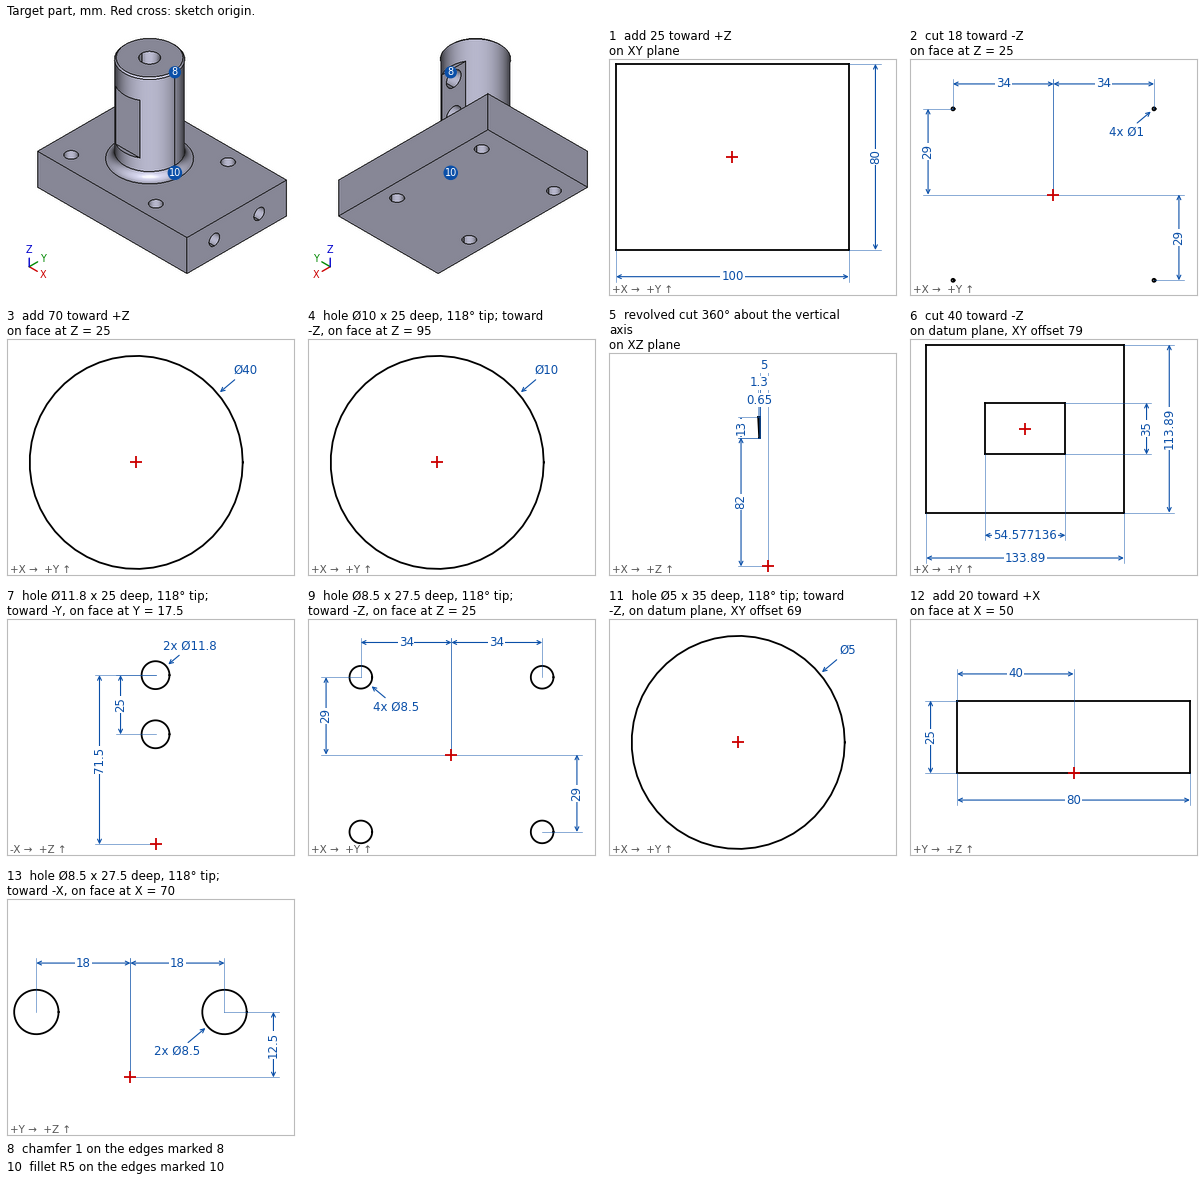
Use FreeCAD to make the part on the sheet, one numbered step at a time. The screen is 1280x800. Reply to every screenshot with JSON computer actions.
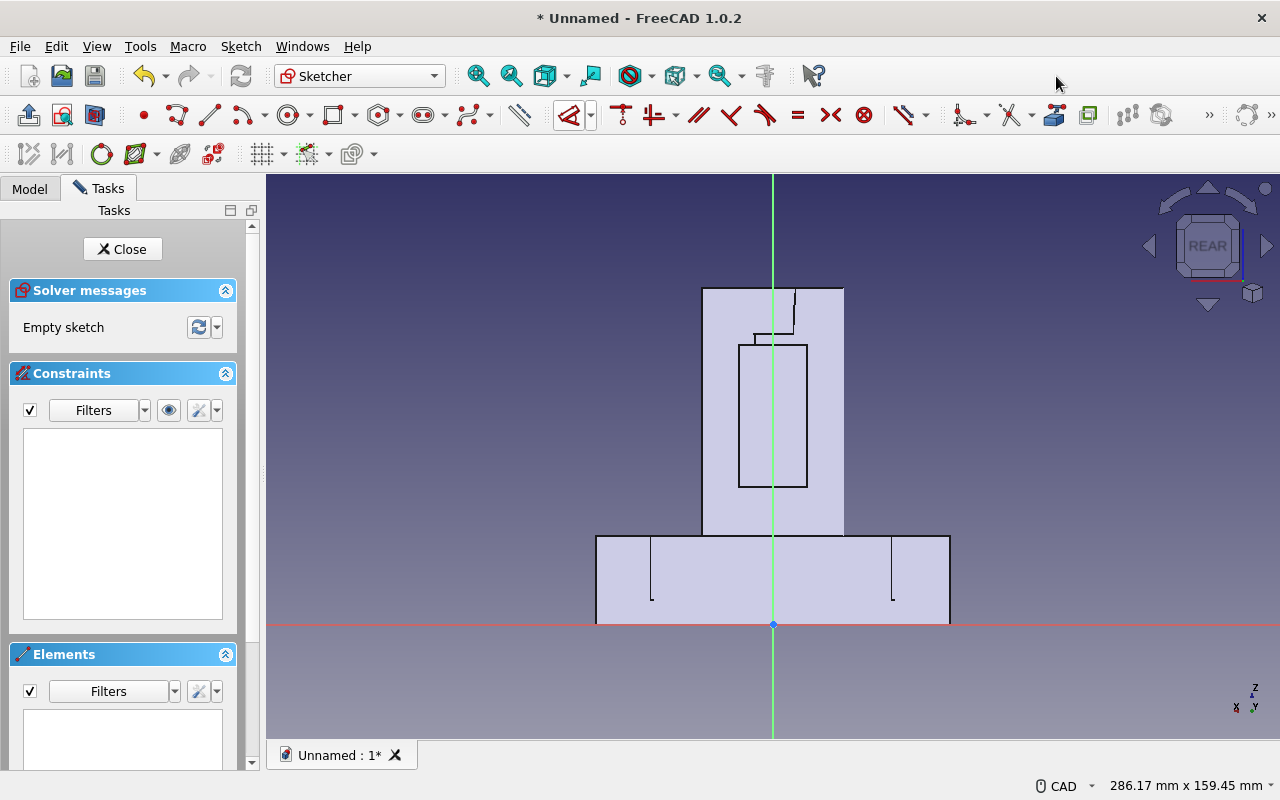
{"action": "key", "text": "g c"}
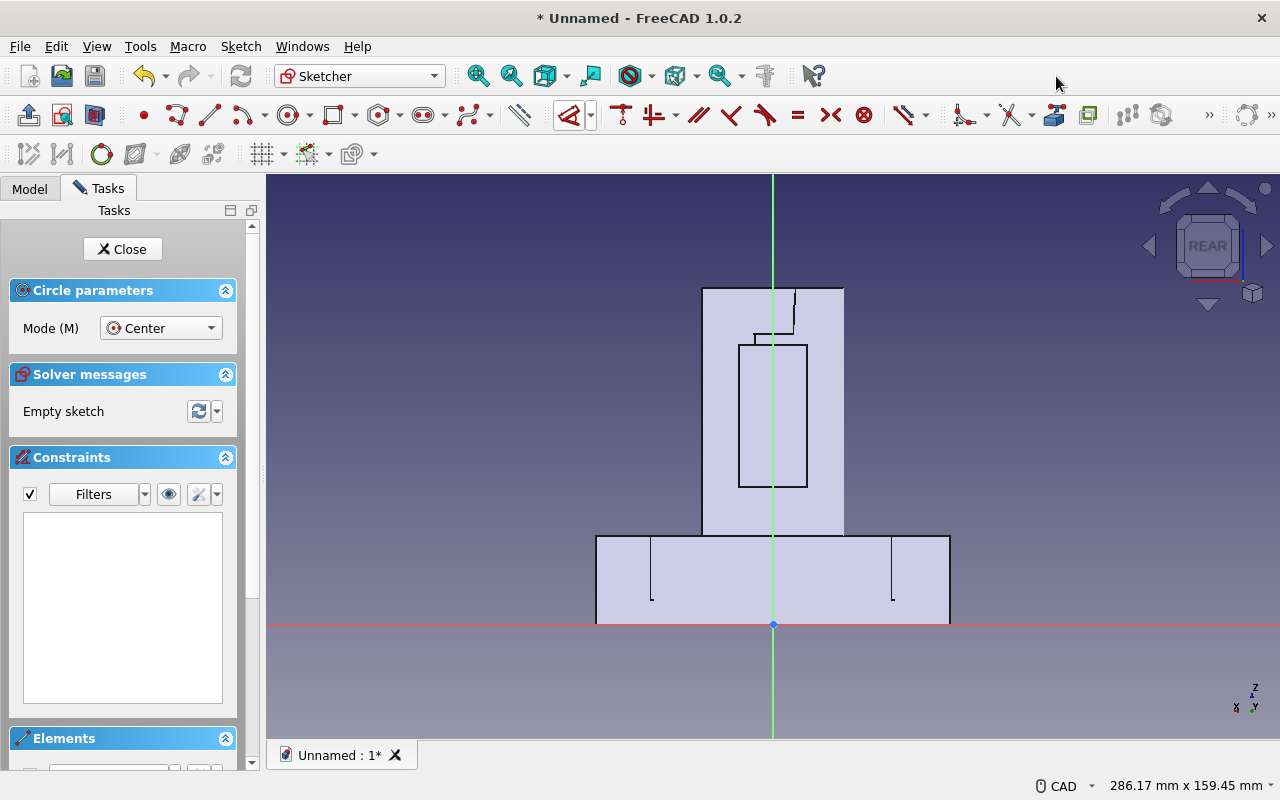
{"action": "left_click", "coordinate": [773, 371]}
{"action": "mouse_move", "coordinate": [788, 357]}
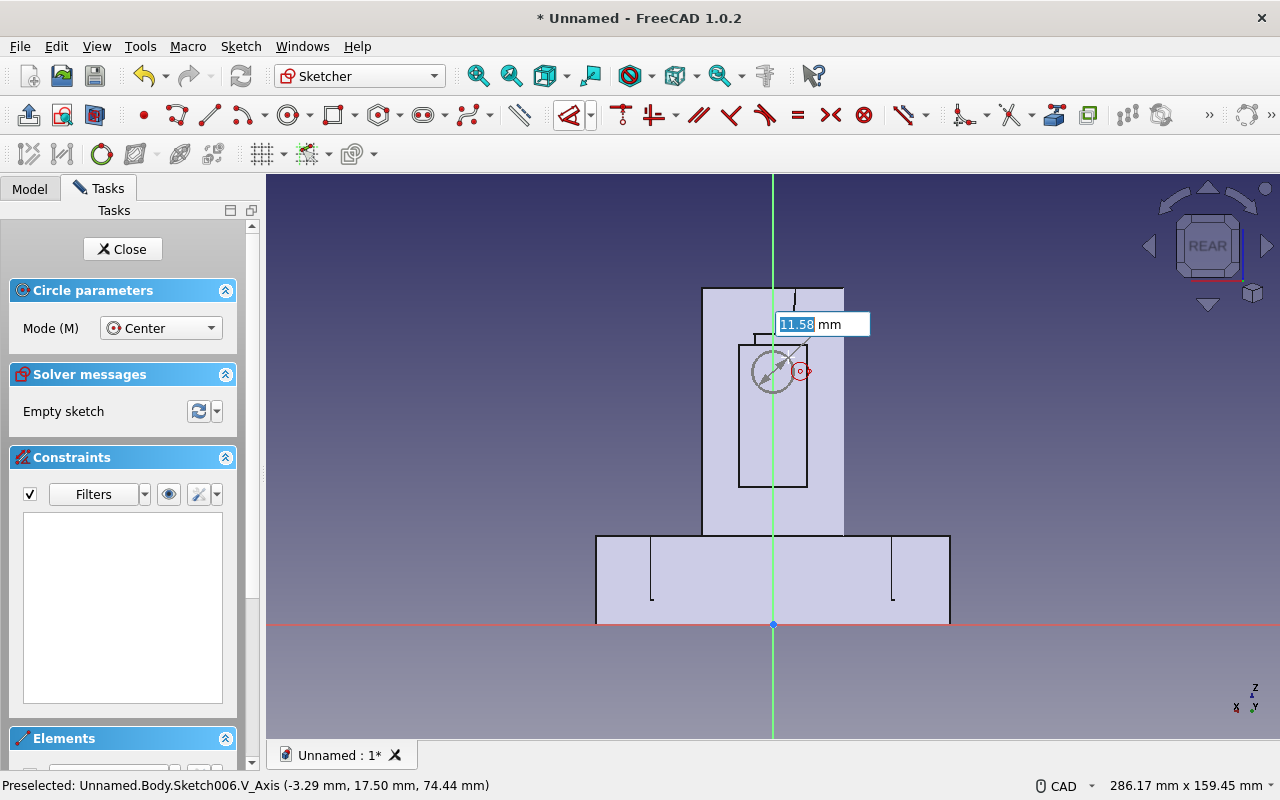
{"action": "type", "text": "11.8"}
{"action": "key", "text": "Return"}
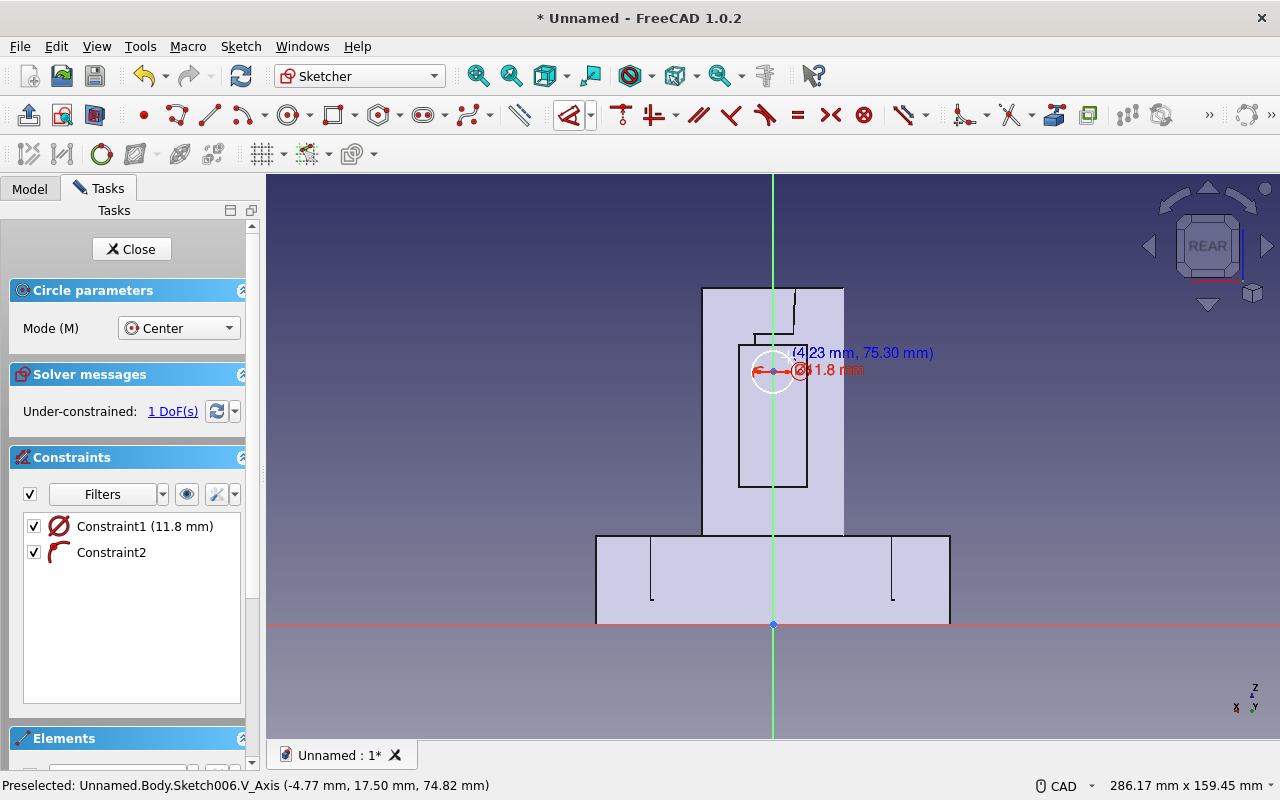
{"action": "left_click", "coordinate": [773, 460]}
{"action": "mouse_move", "coordinate": [788, 445]}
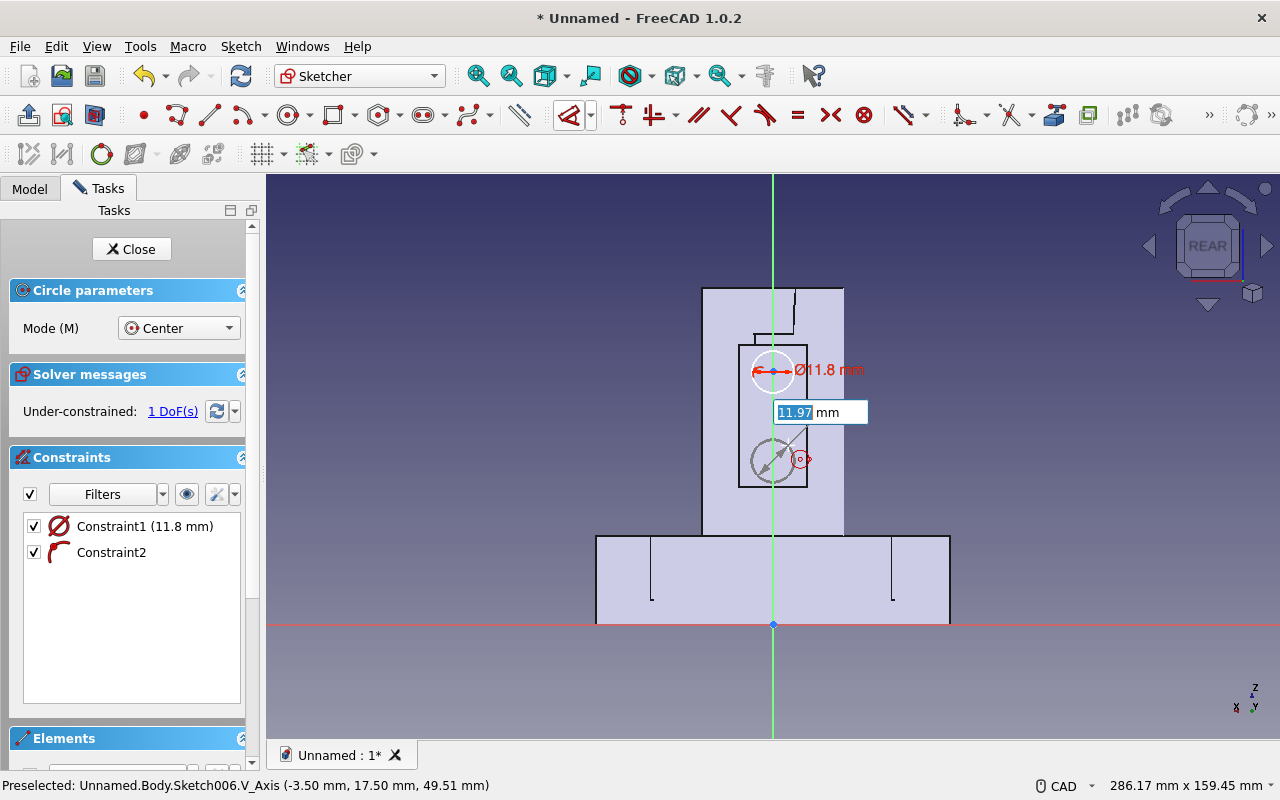
{"action": "type", "text": "11.8"}
{"action": "key", "text": "Return"}
{"action": "key", "text": "Escape"}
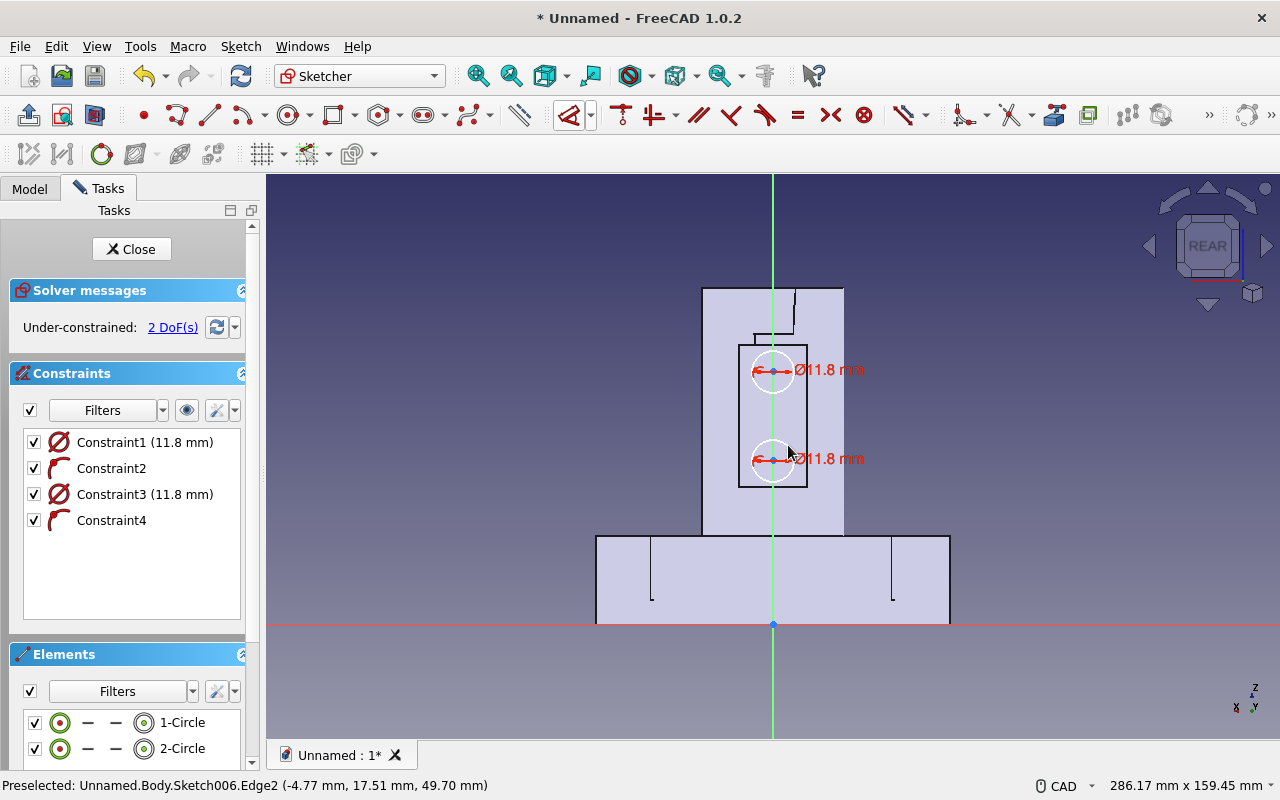
{"action": "left_click", "coordinate": [773, 372]}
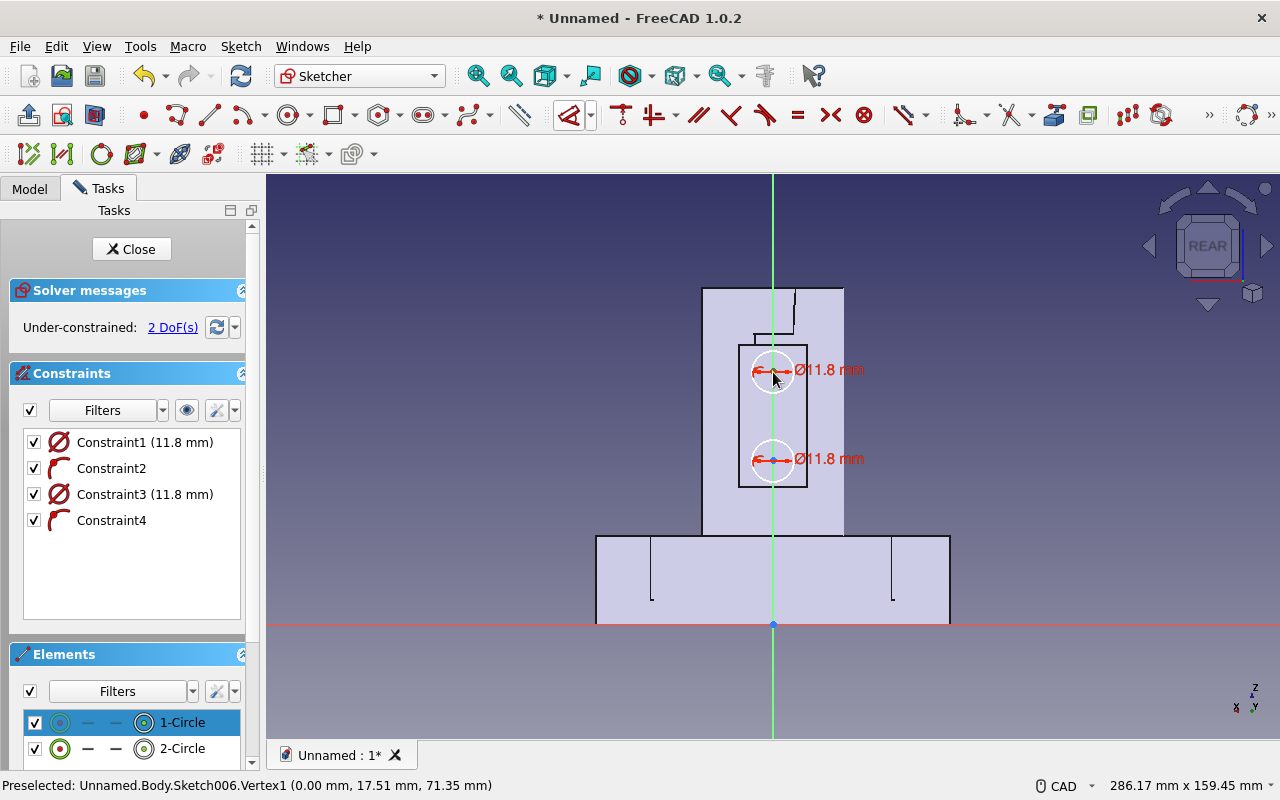
{"action": "left_click", "coordinate": [773, 461]}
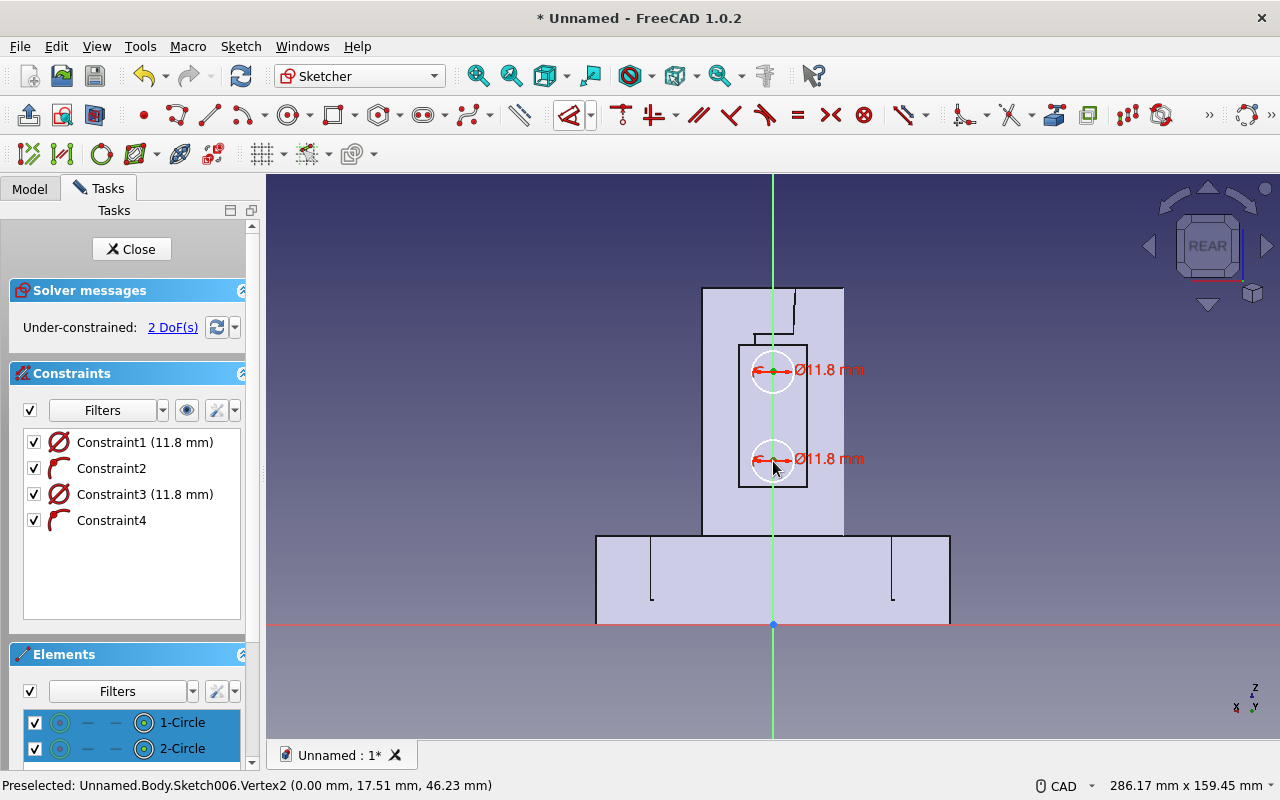
{"action": "left_click", "coordinate": [590, 116]}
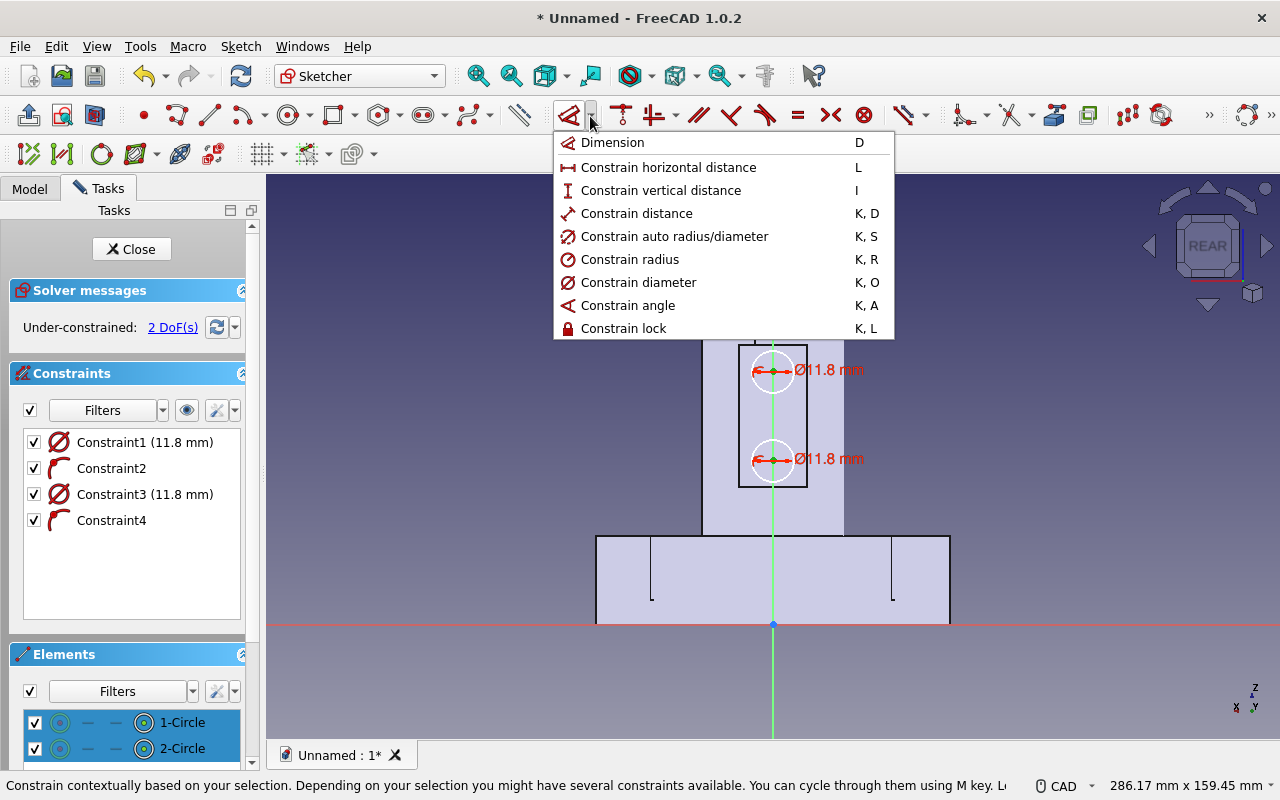
{"action": "left_click", "coordinate": [724, 190]}